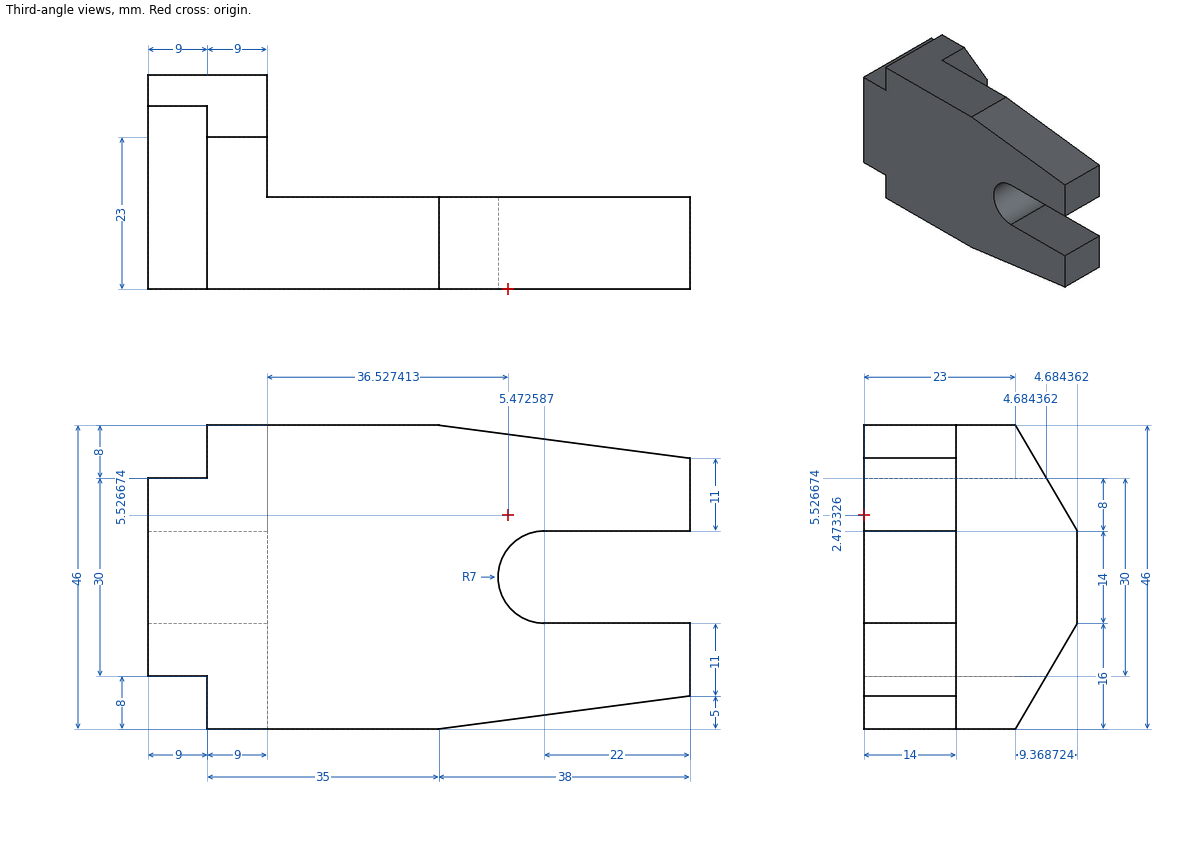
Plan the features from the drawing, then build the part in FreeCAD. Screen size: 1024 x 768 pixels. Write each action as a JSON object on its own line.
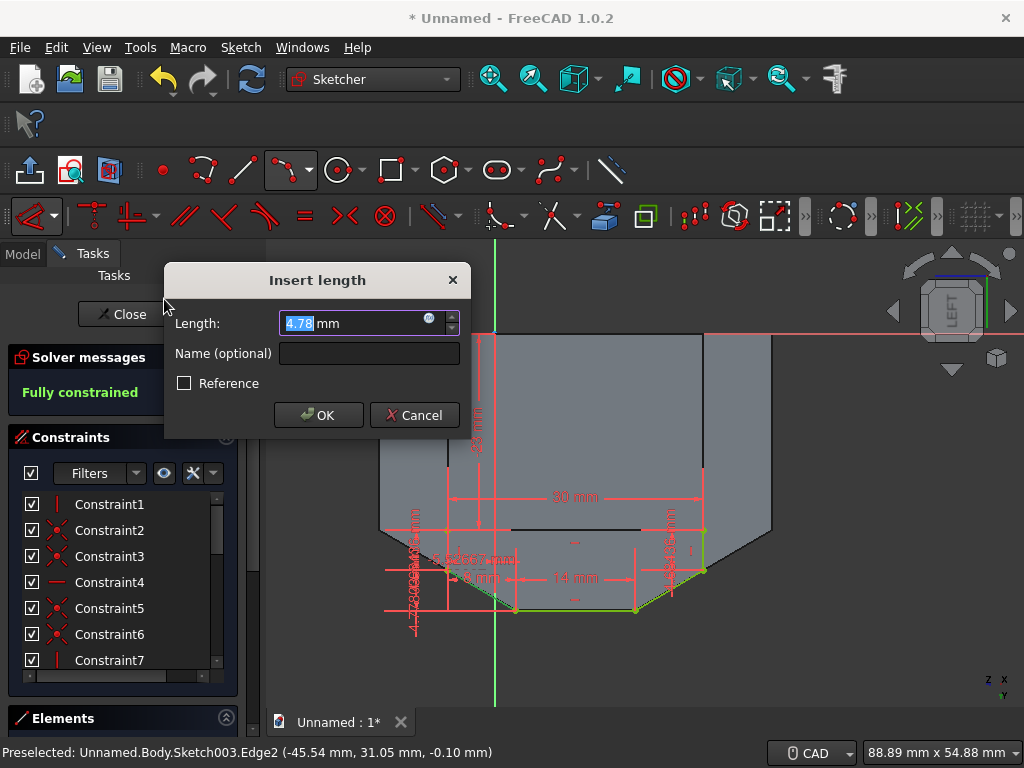
{"action": "type", "text": "4.684362"}
{"action": "key", "text": "Return"}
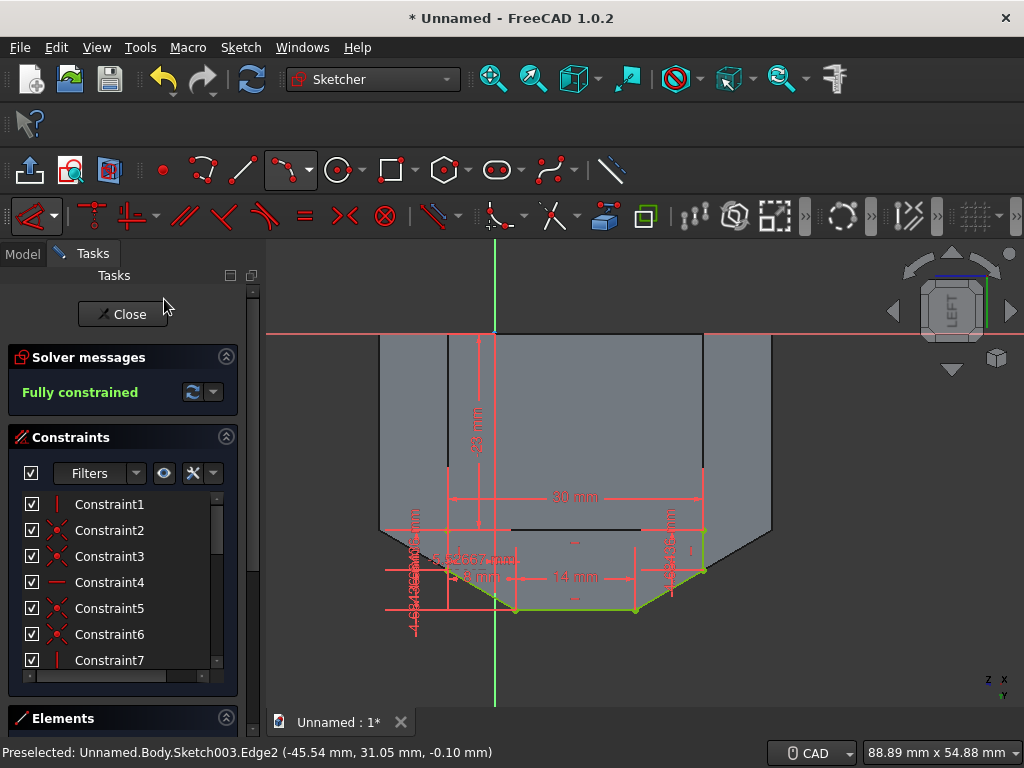
{"action": "left_click", "coordinate": [123, 314]}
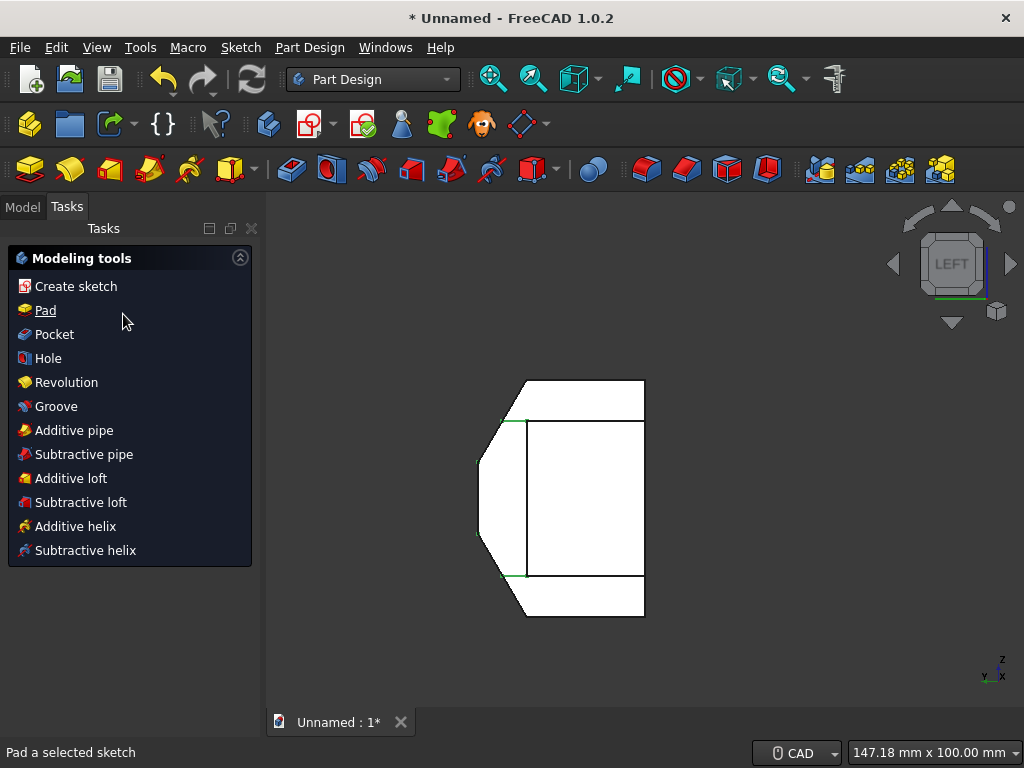
{"action": "left_click", "coordinate": [30, 170]}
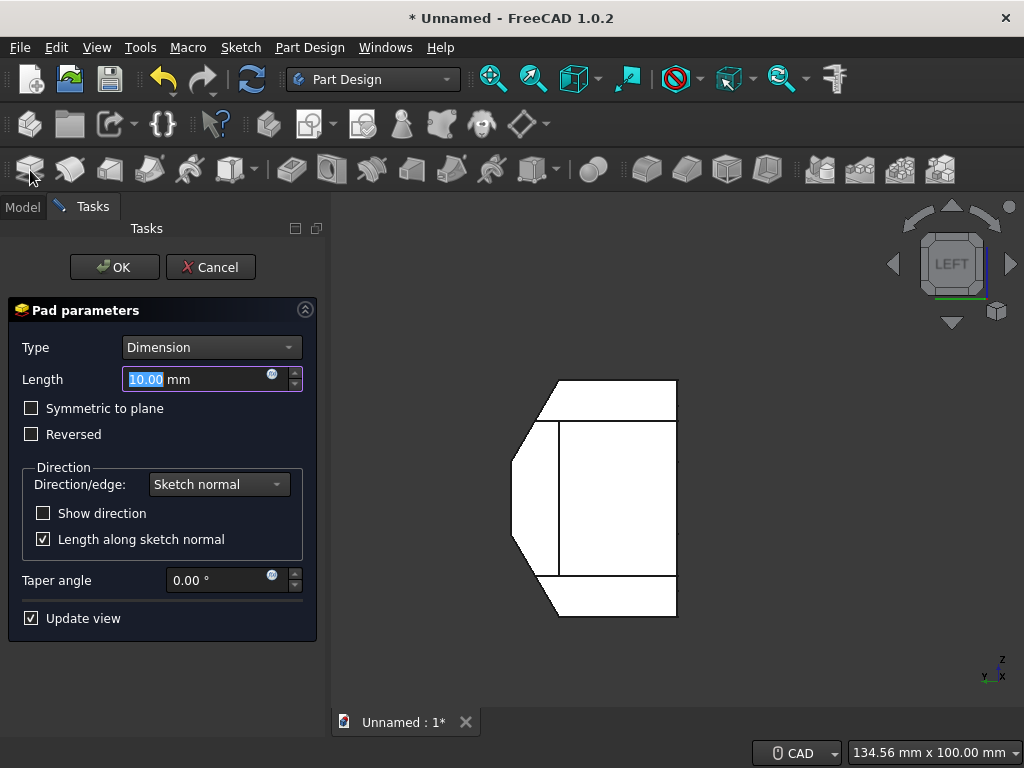
{"action": "type", "text": "9"}
{"action": "key", "text": "Tab"}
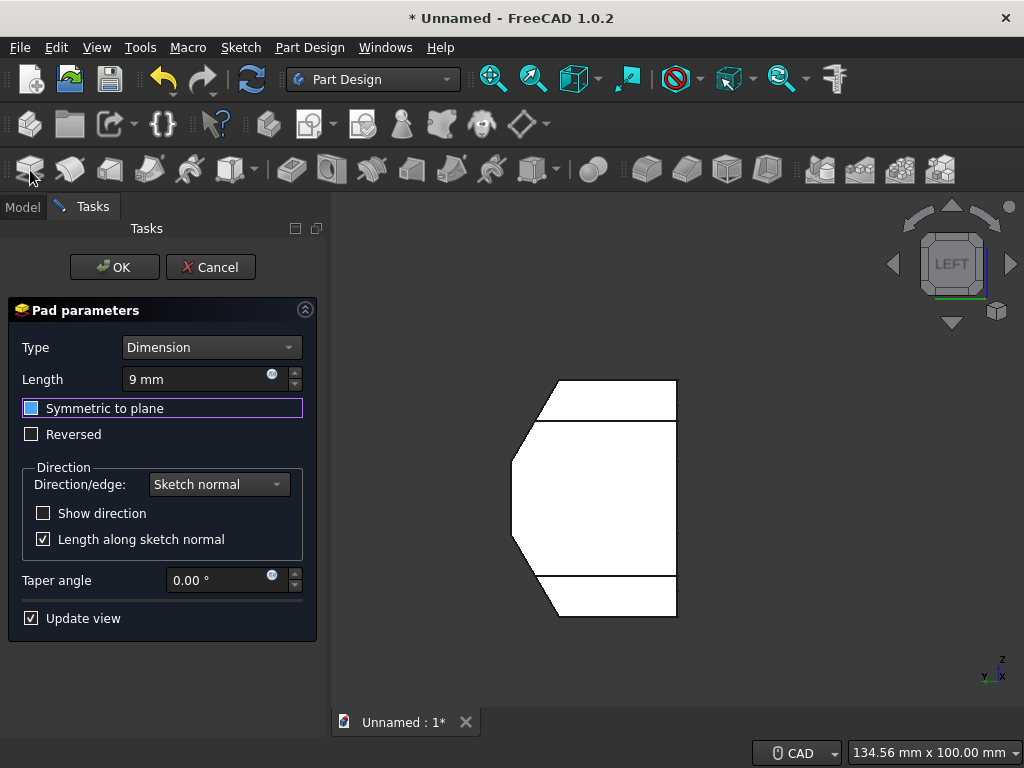
{"action": "left_click", "coordinate": [115, 267]}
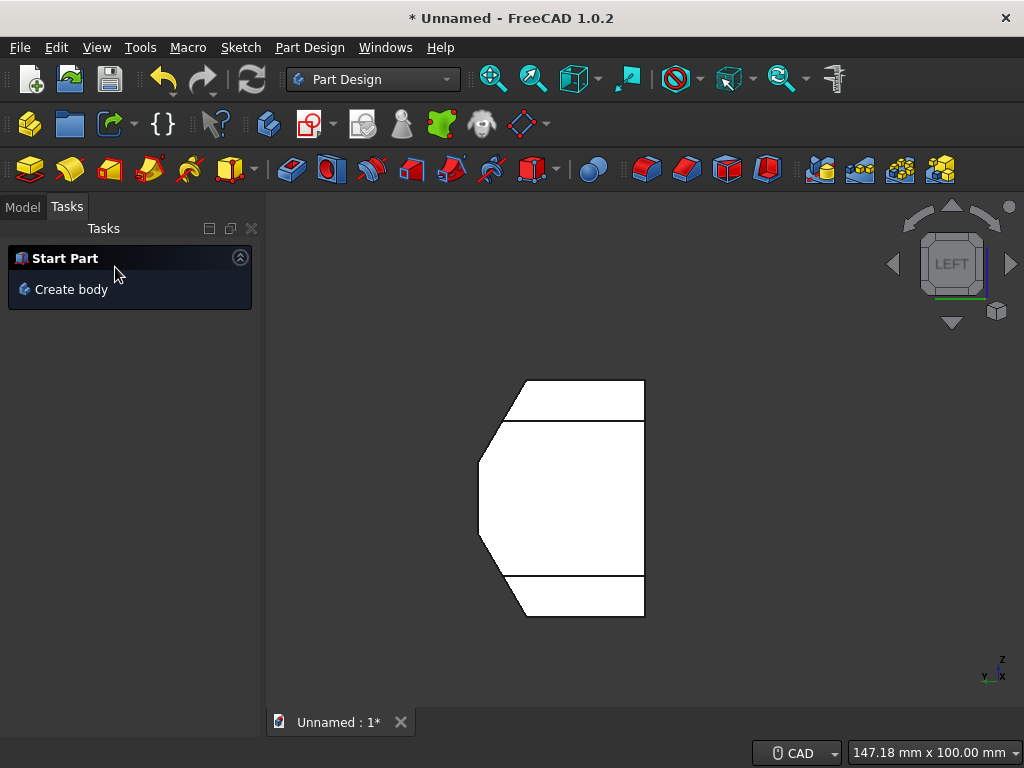
{"action": "key", "text": "0"}